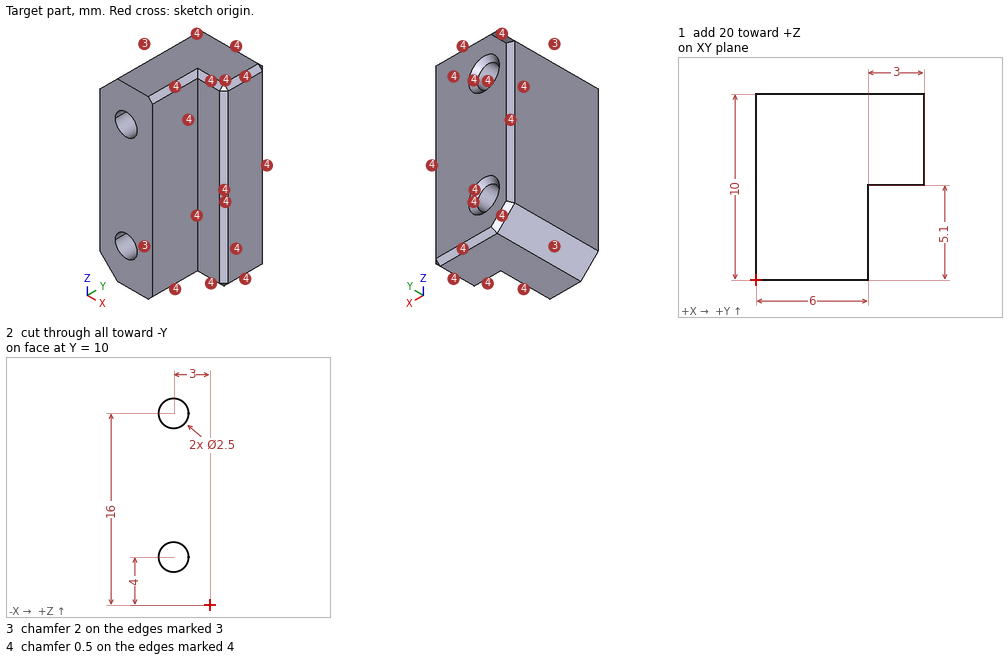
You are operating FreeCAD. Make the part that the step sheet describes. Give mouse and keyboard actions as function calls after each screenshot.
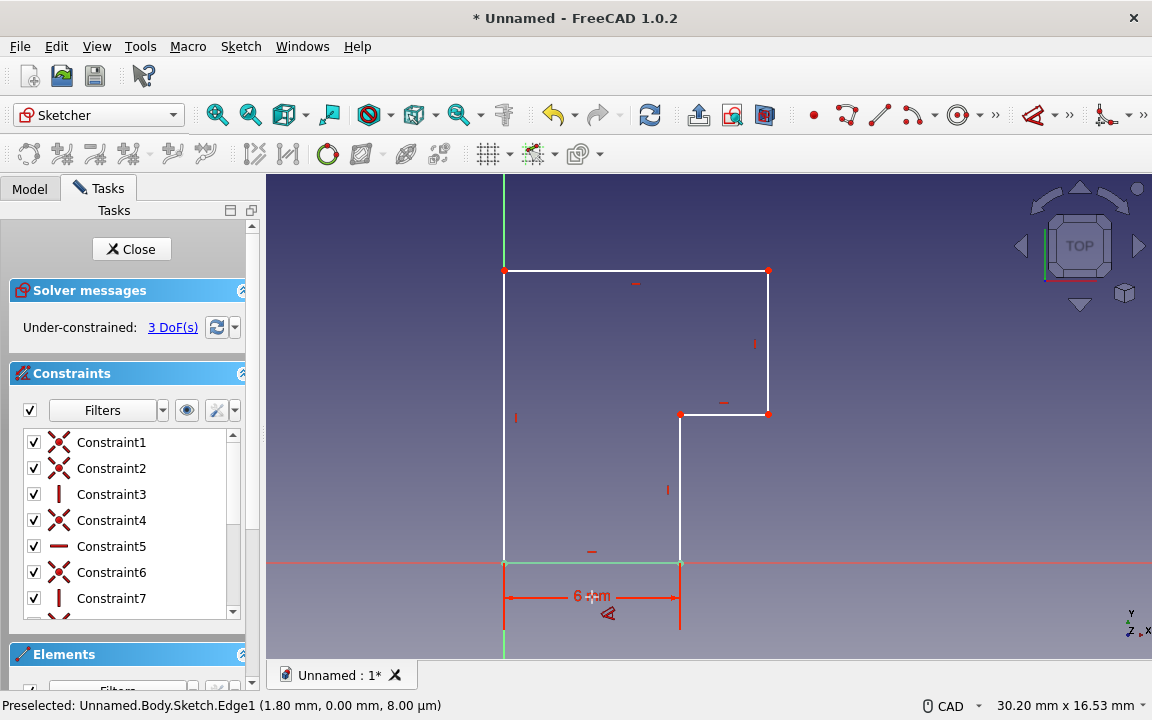
click(707, 415)
click(724, 381)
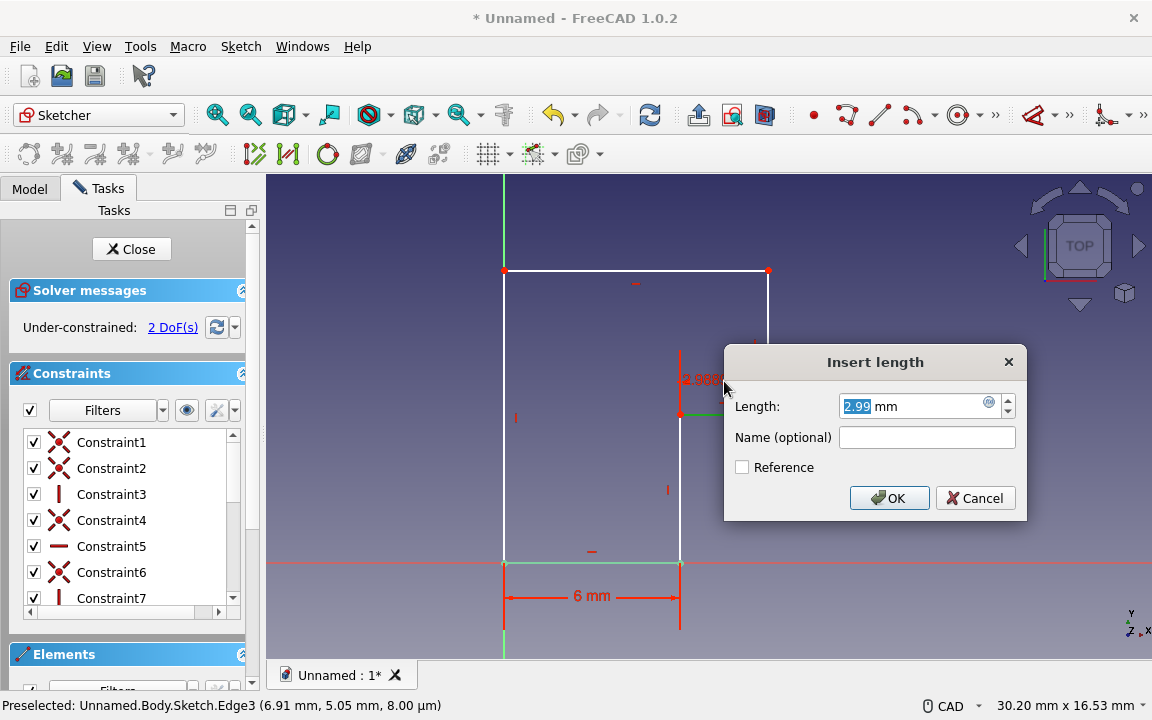
text(3)
key(Return)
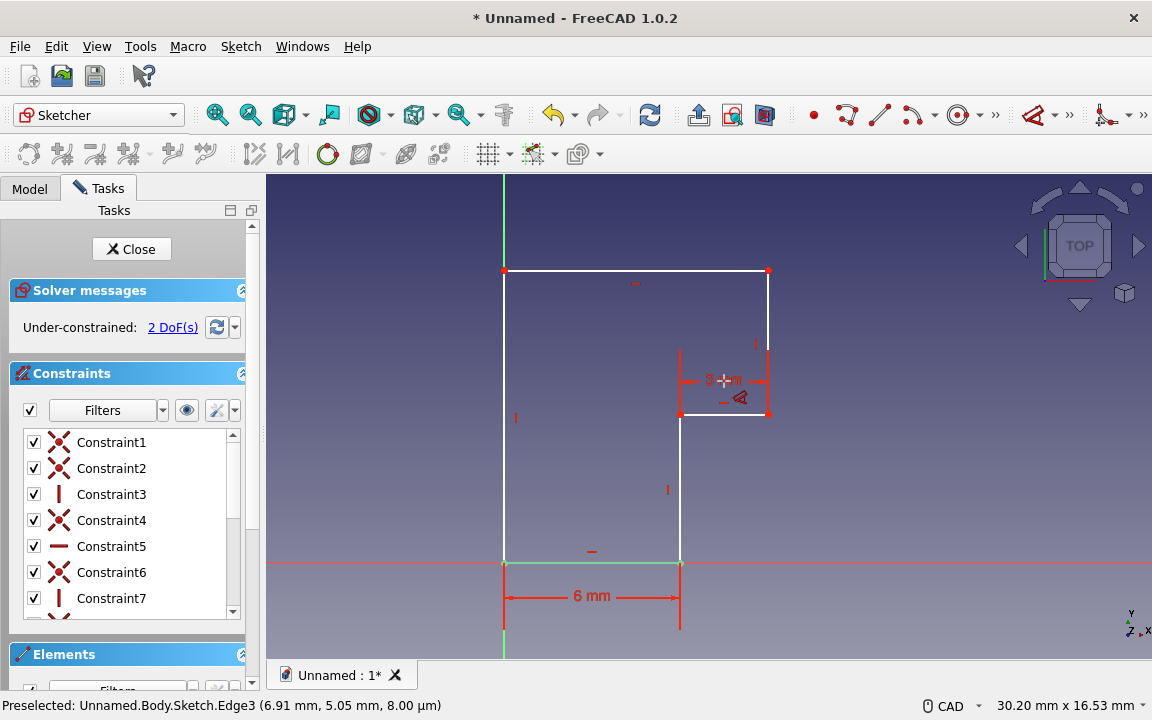
click(504, 359)
click(470, 417)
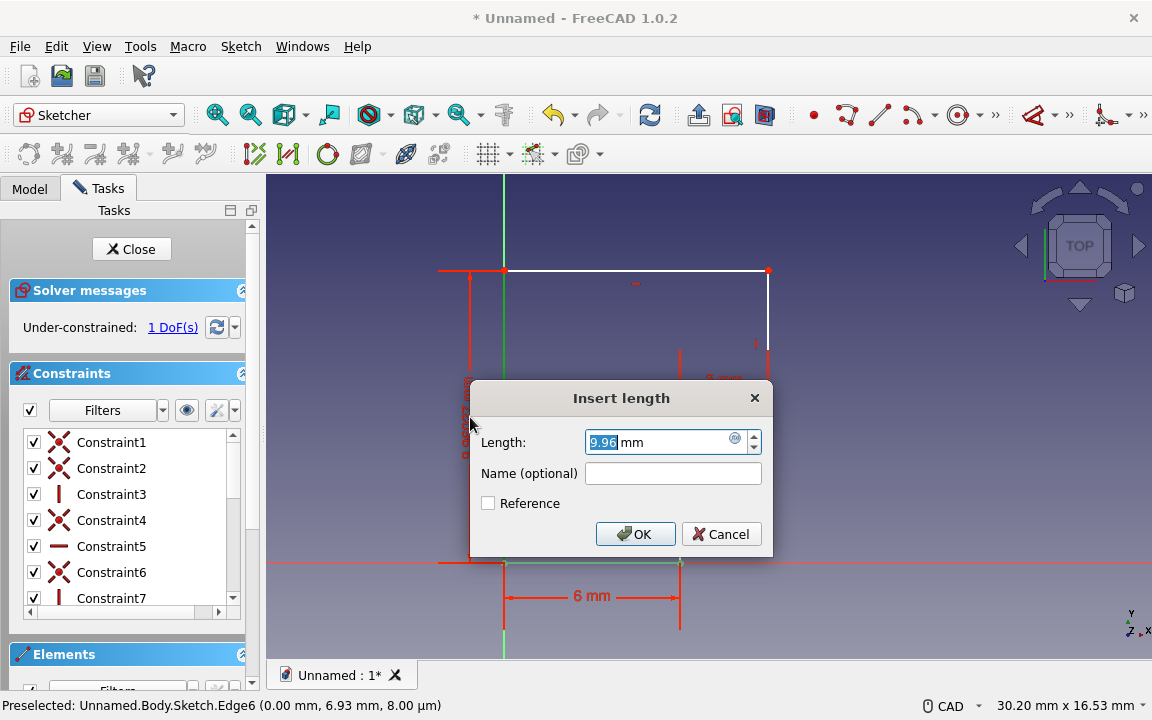
text(10)
key(Return)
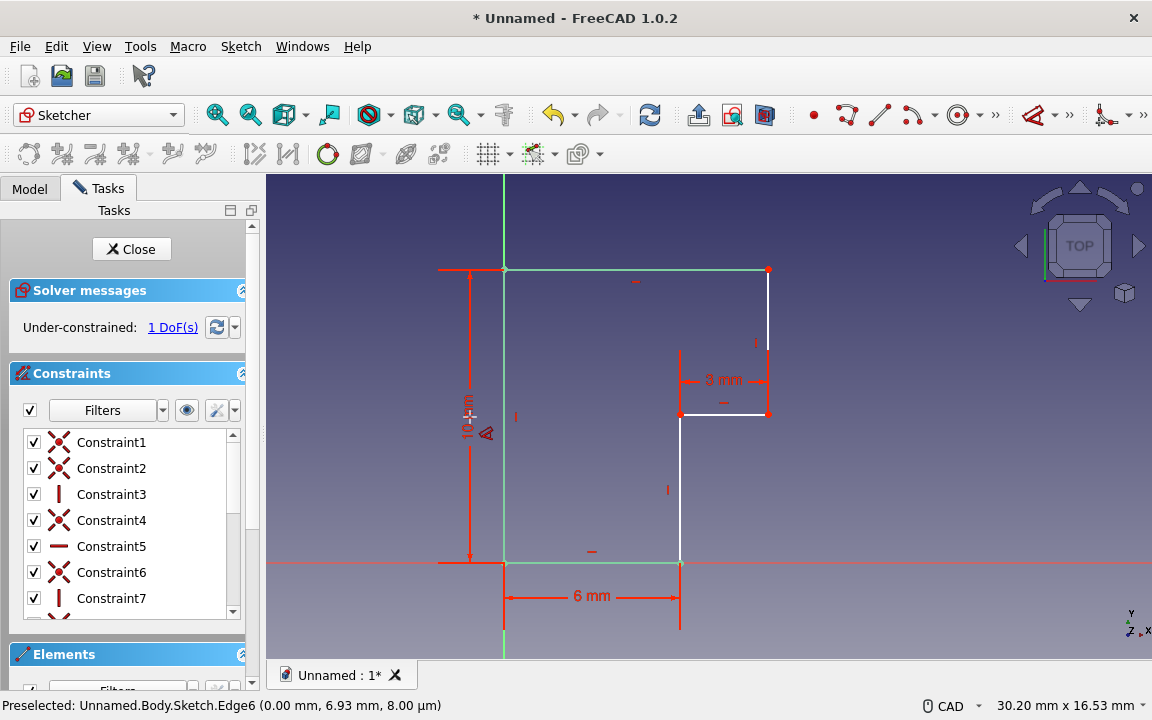
click(680, 519)
click(714, 489)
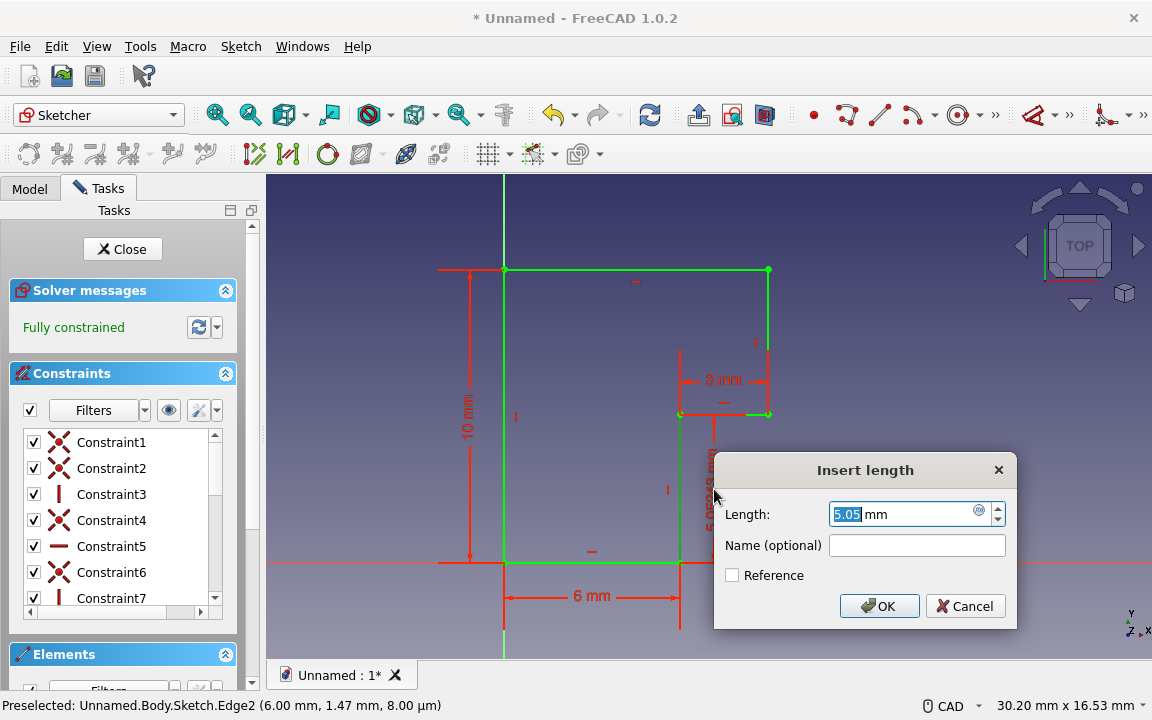
text(5.1)
key(Return)
key(Escape)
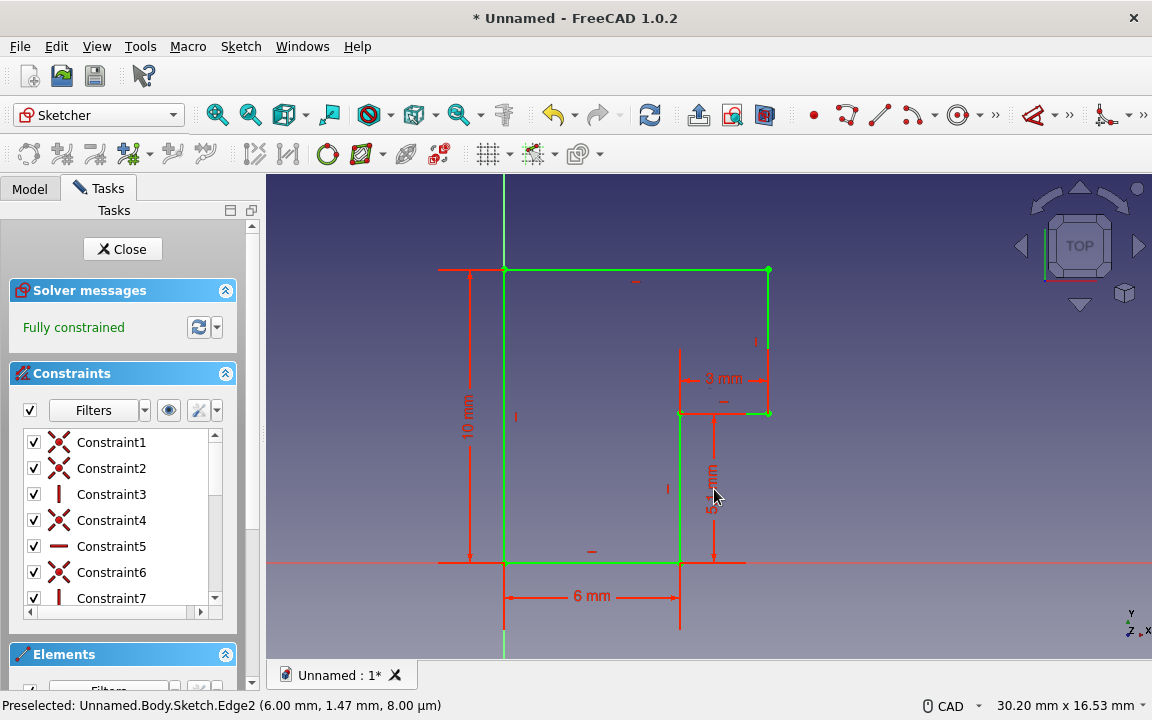
click(123, 249)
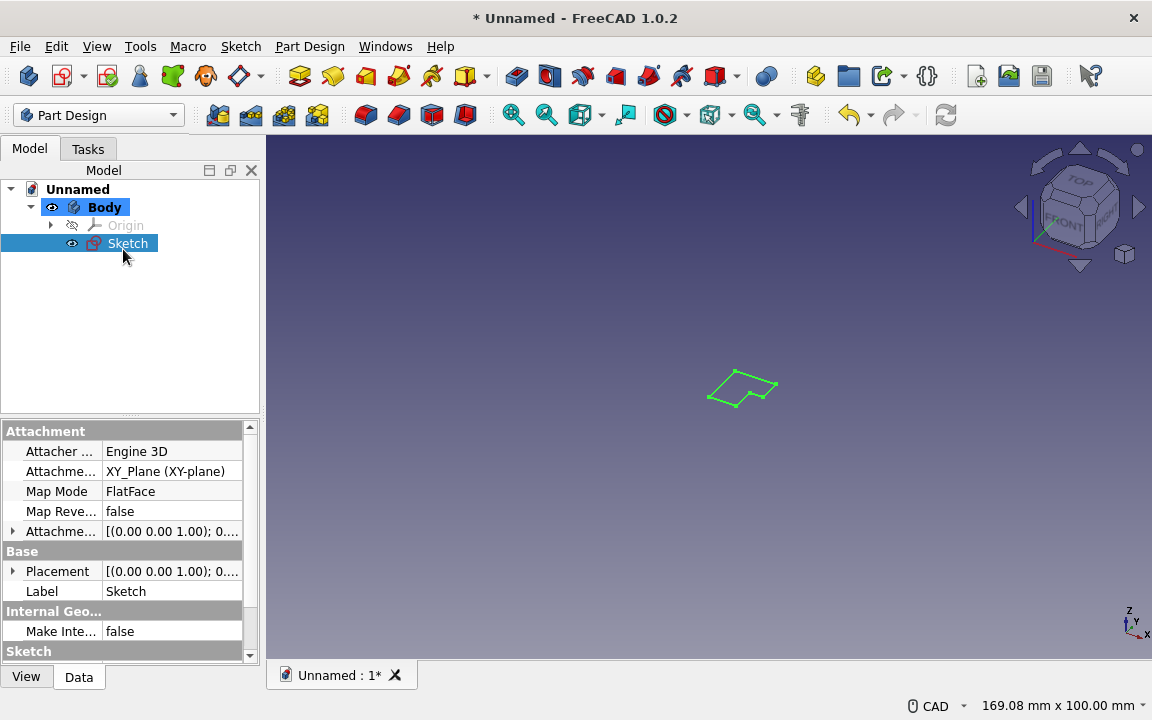
click(300, 76)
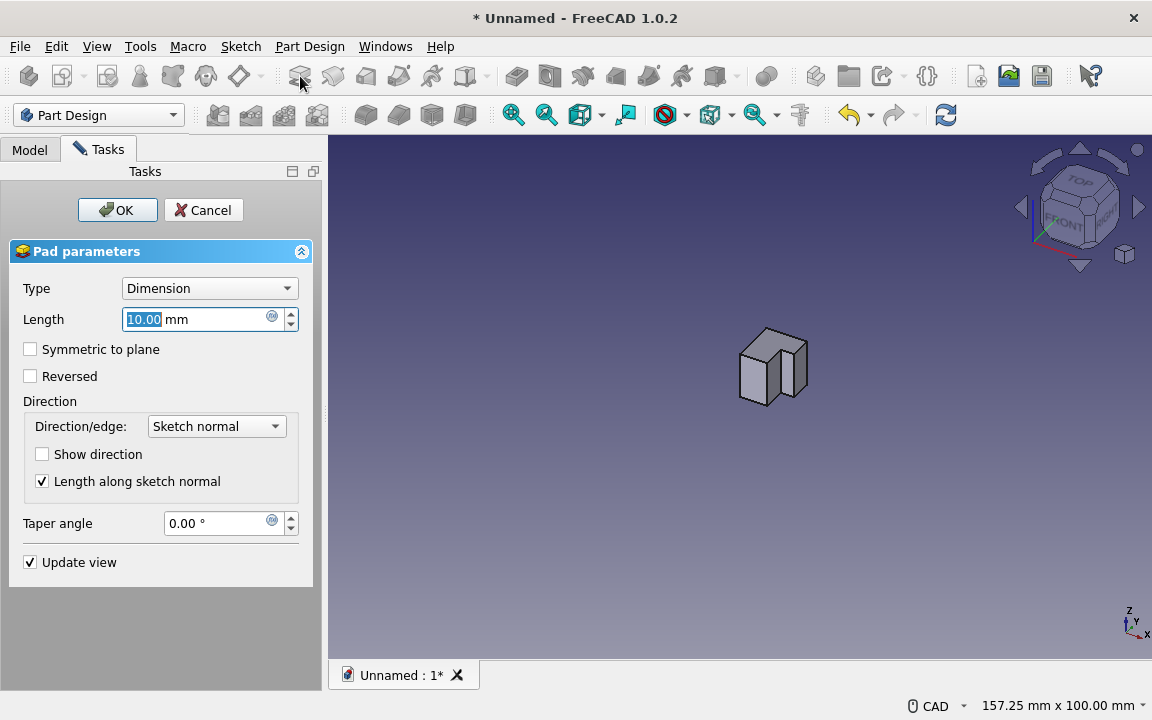
text(20)
key(Tab)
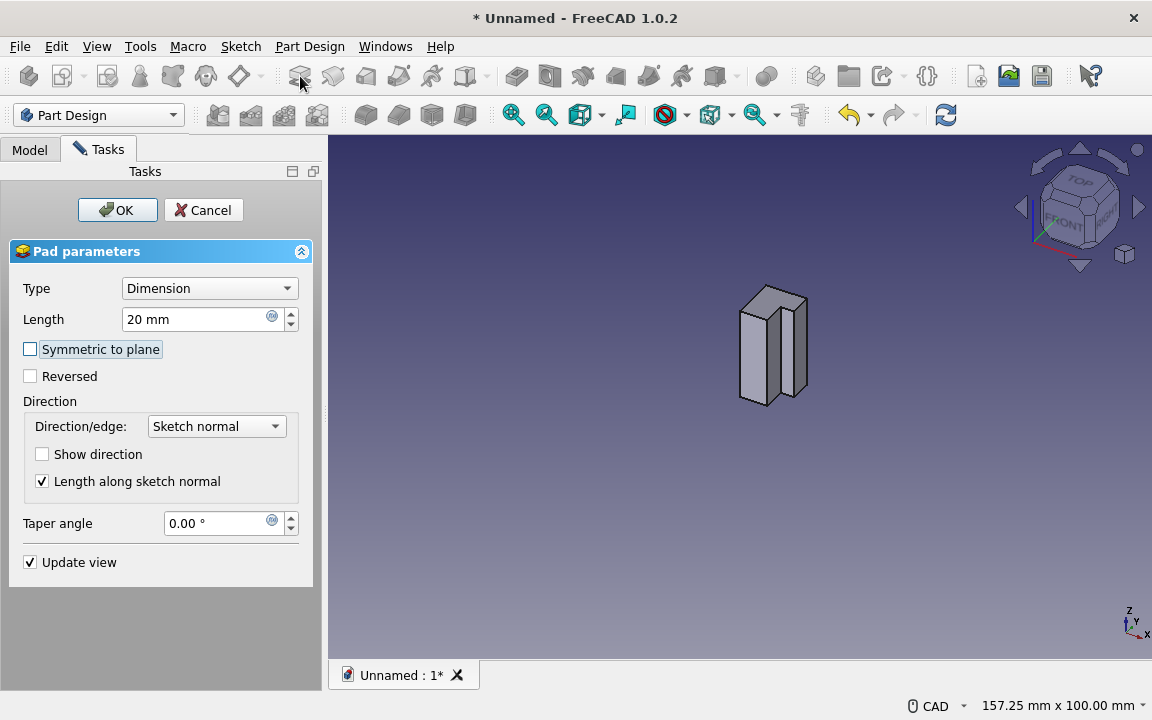
click(118, 210)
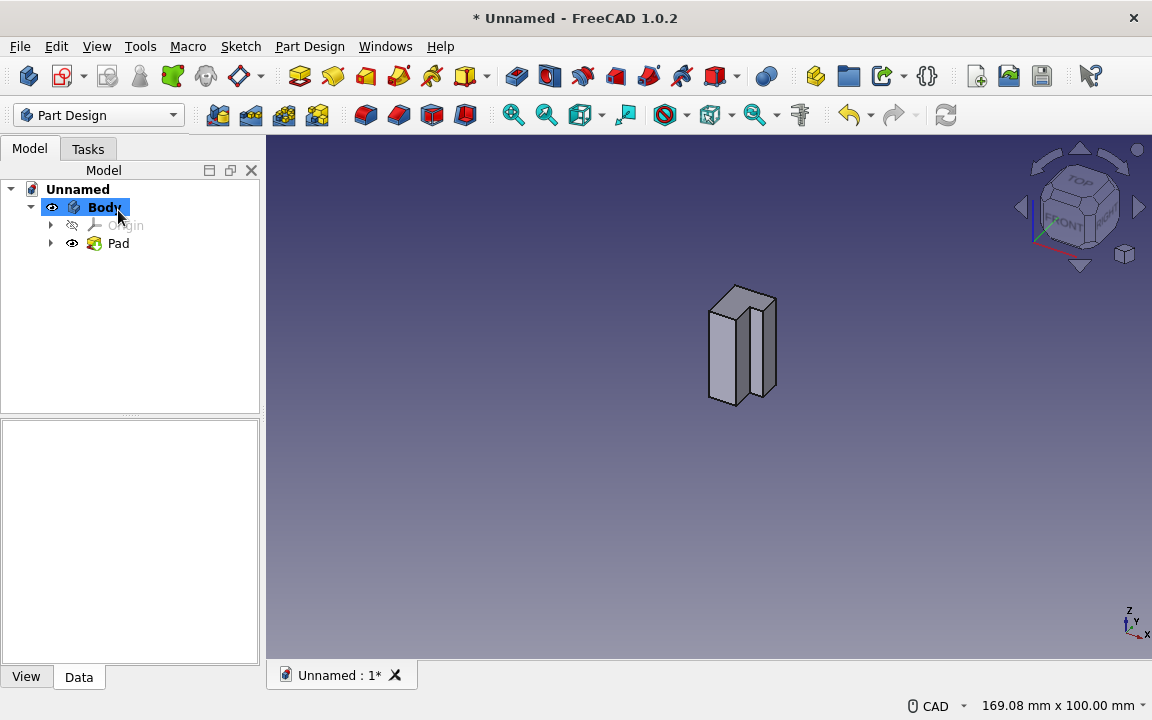
click(514, 116)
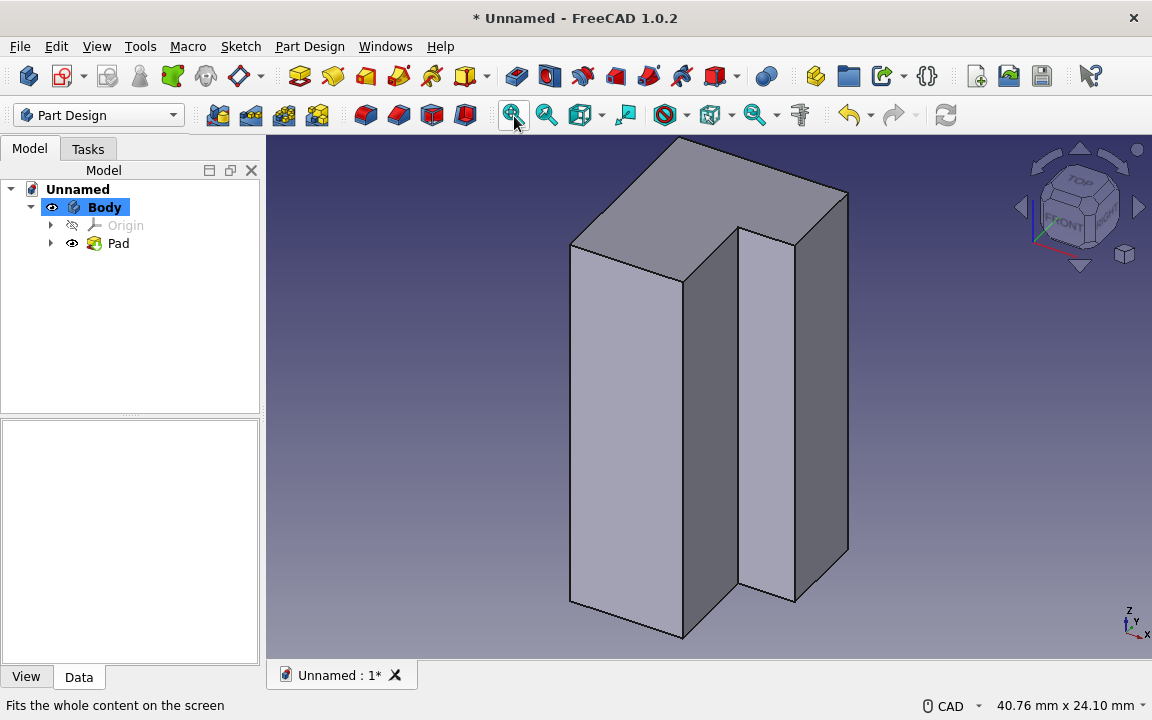
key(4)